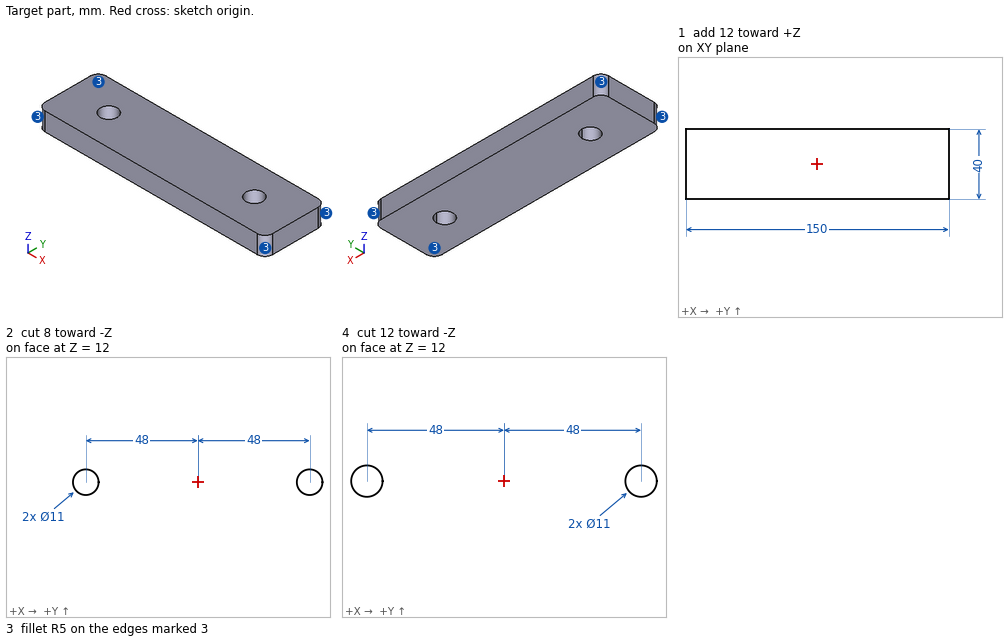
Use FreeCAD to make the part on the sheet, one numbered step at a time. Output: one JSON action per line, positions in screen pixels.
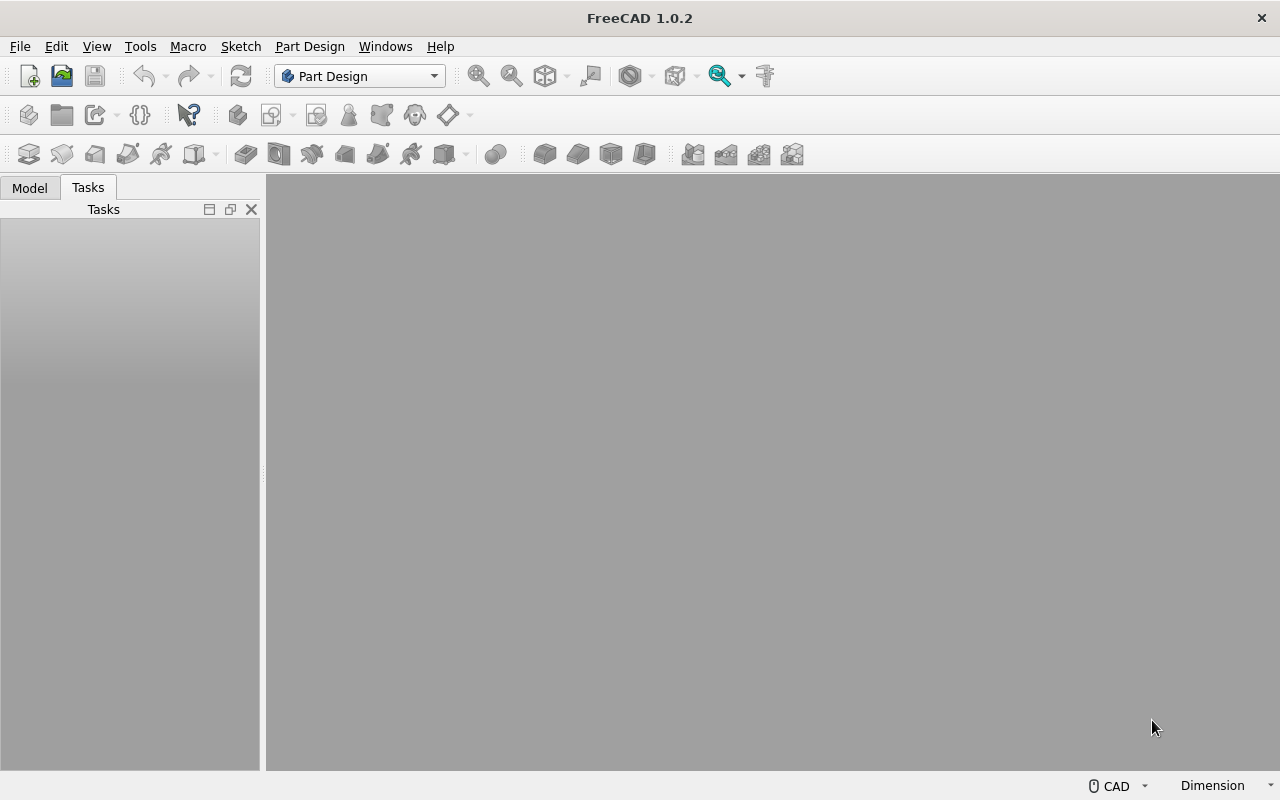
{"action": "left_click", "coordinate": [29, 76]}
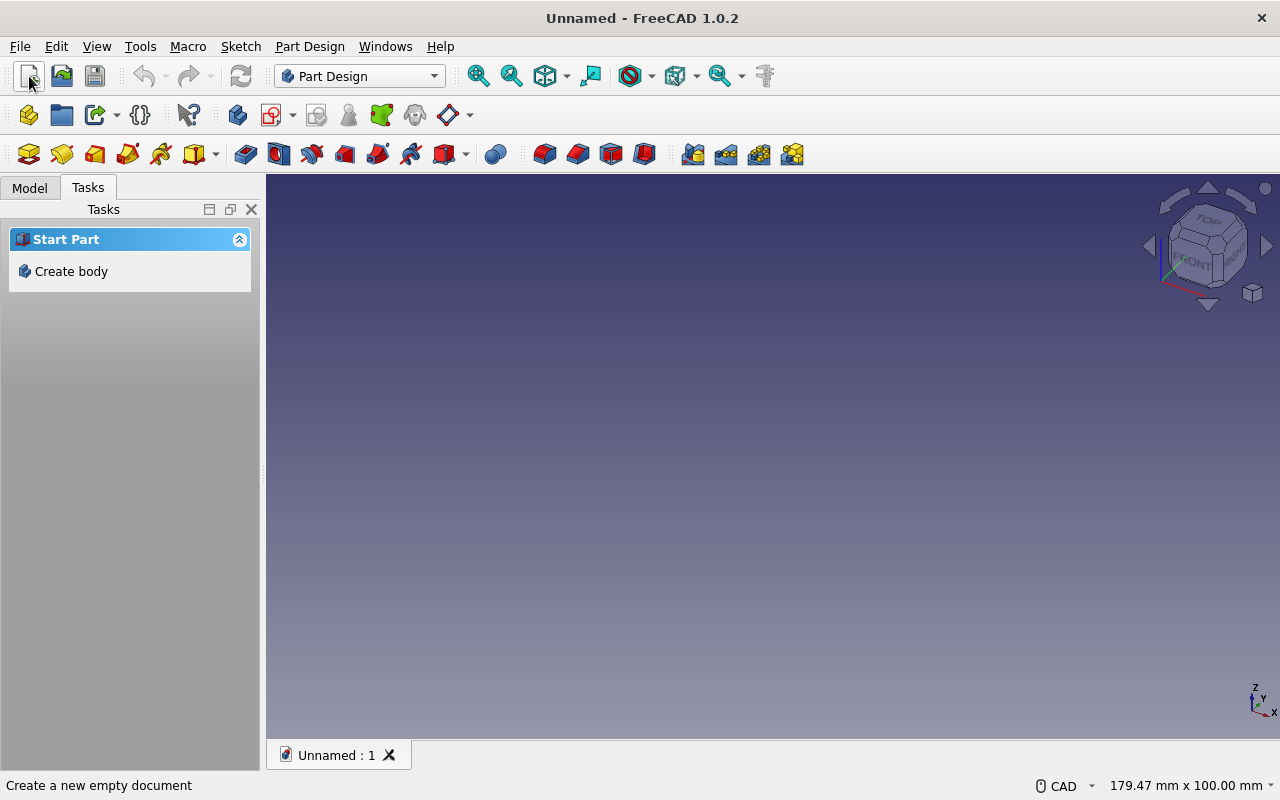
{"action": "left_click", "coordinate": [270, 116]}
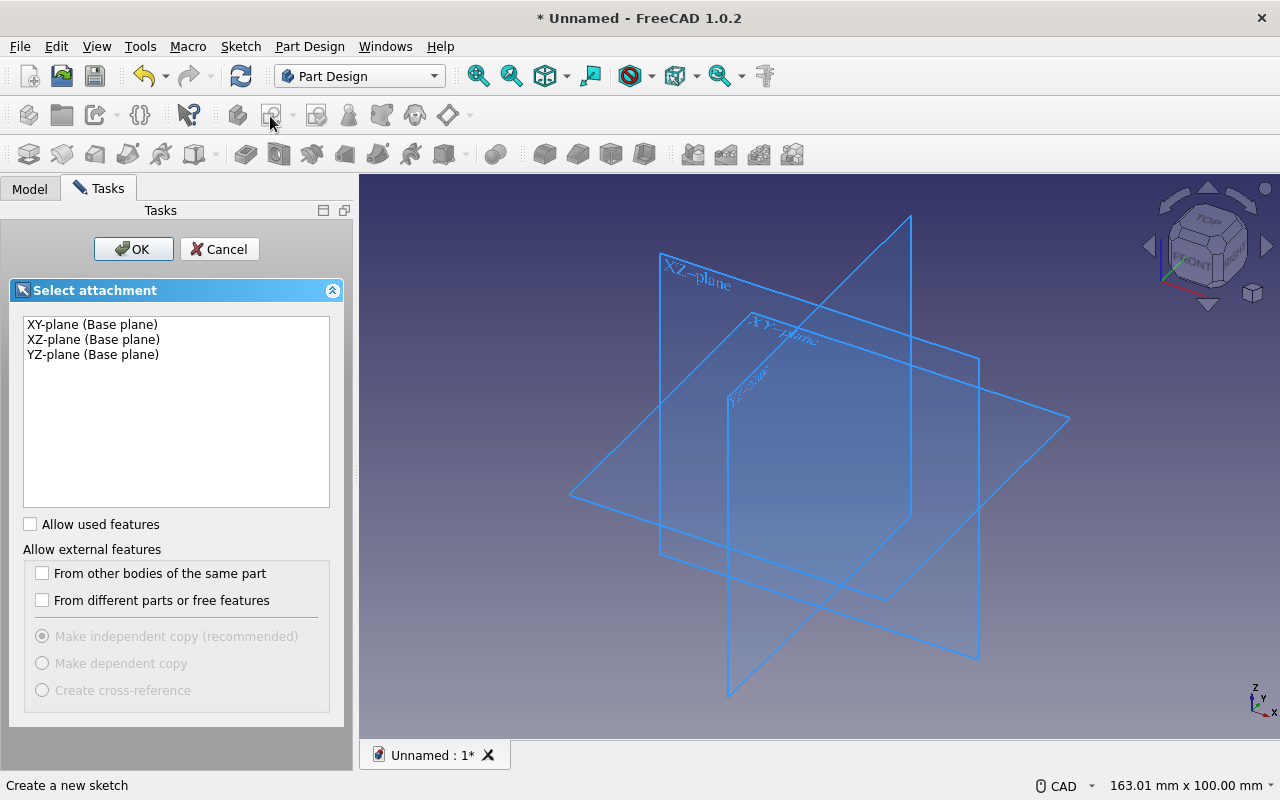
{"action": "left_click", "coordinate": [84, 324]}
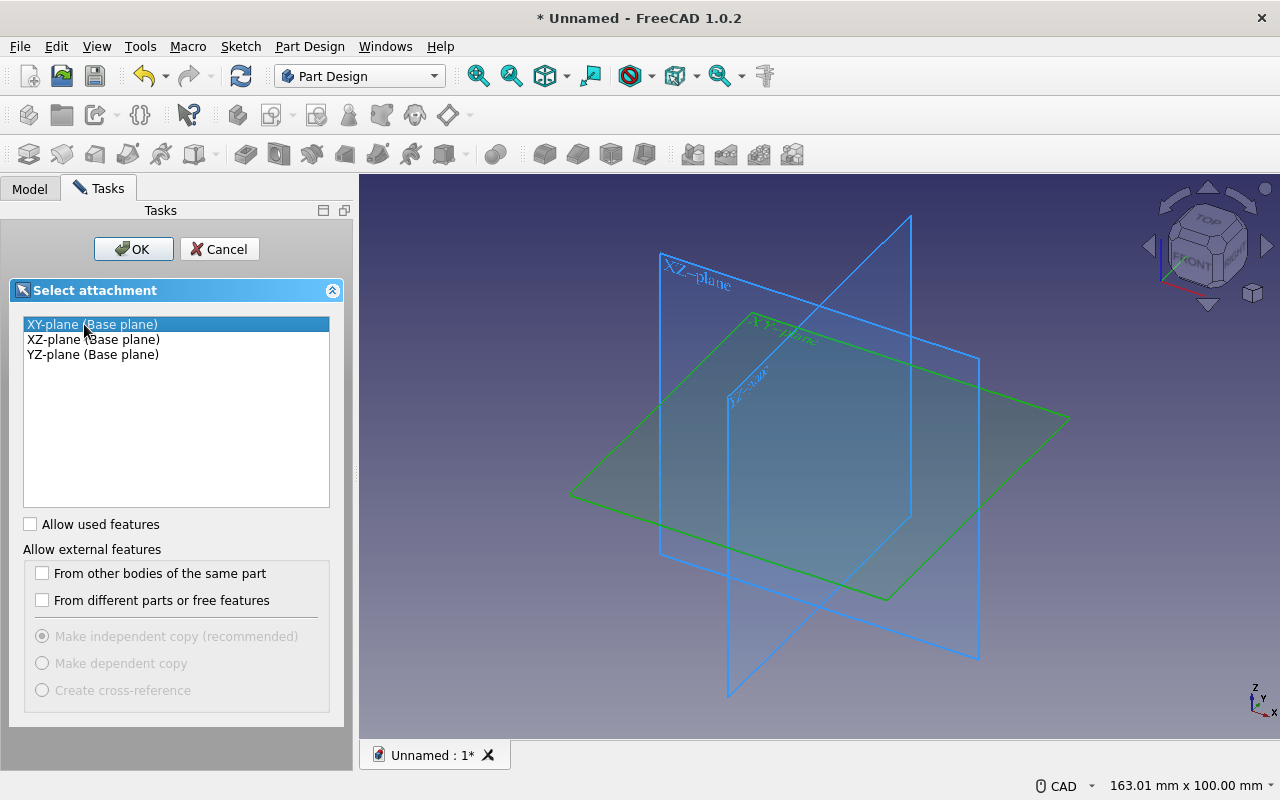
{"action": "left_click", "coordinate": [134, 249]}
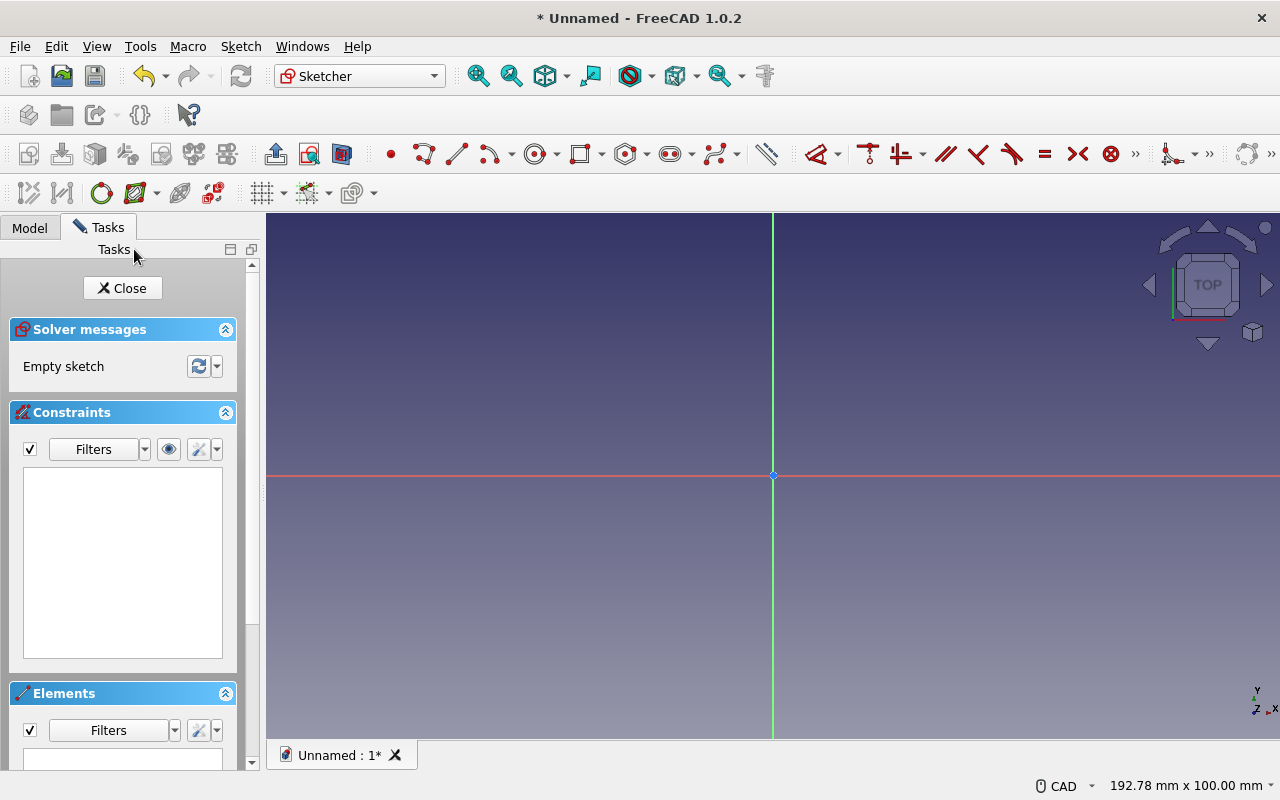
{"action": "scroll", "coordinate": [565, 476], "scroll_direction": "down", "scroll_amount": 2}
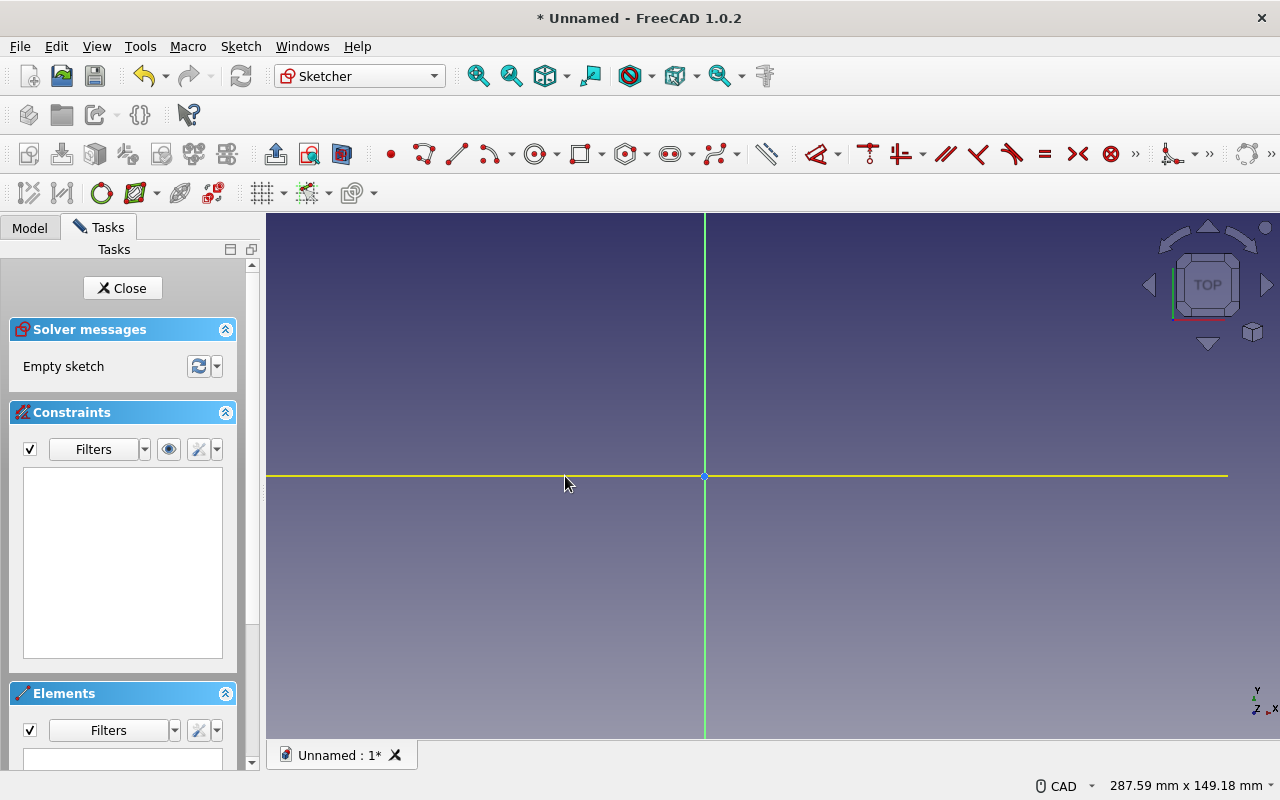
{"action": "left_click", "coordinate": [602, 154]}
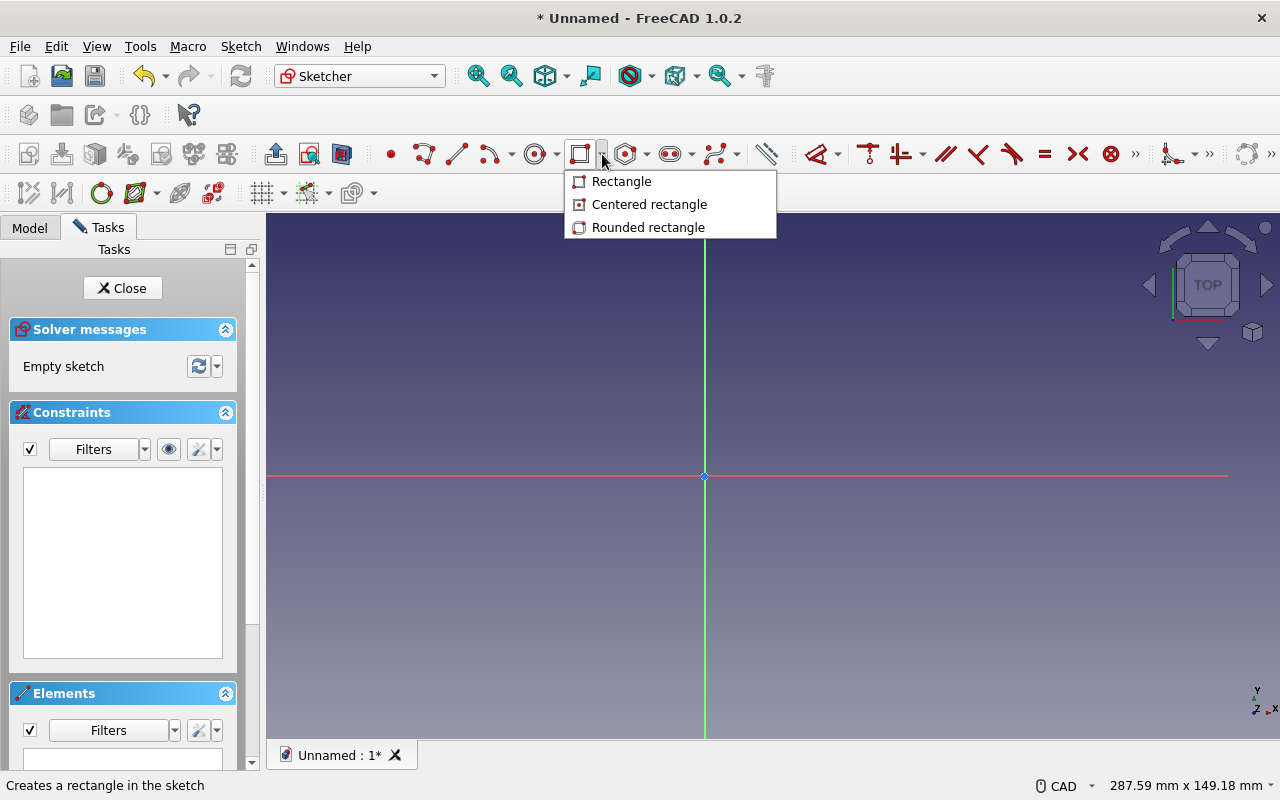
{"action": "left_click", "coordinate": [670, 204]}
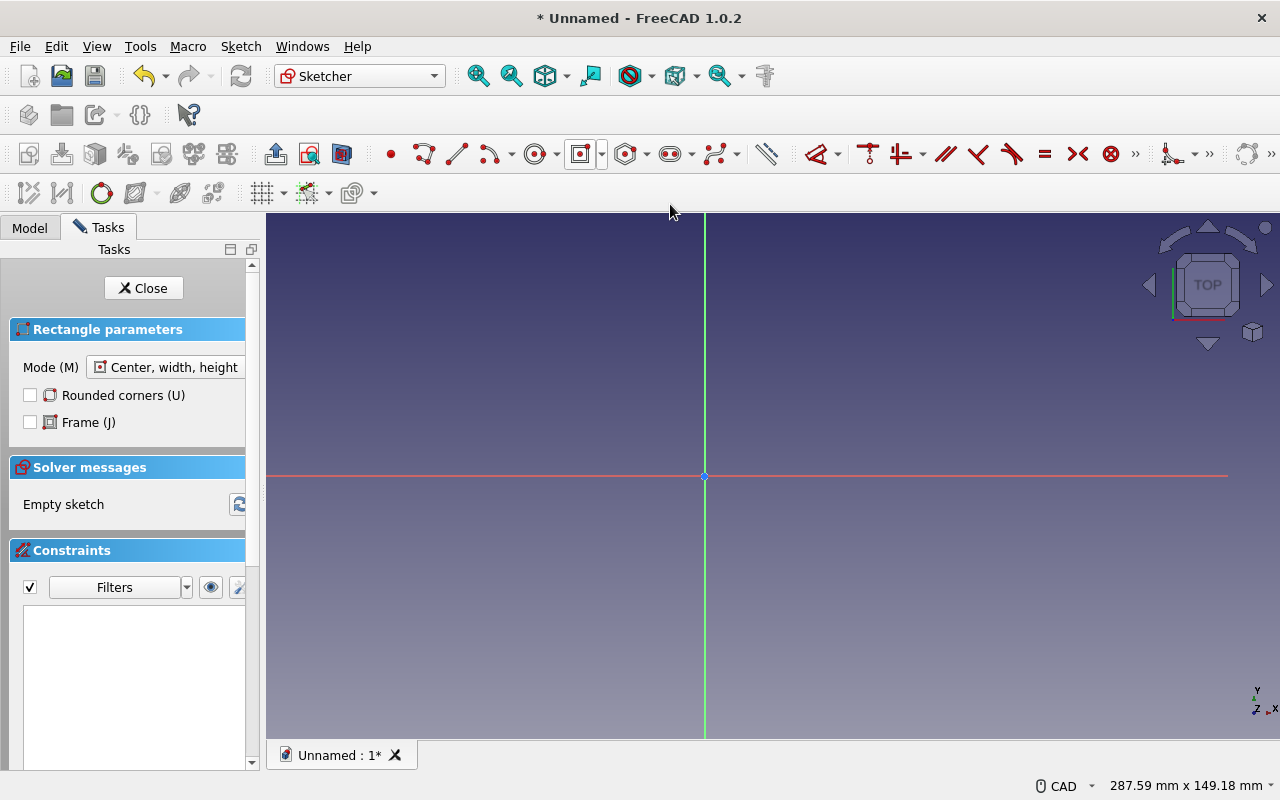
{"action": "left_click", "coordinate": [705, 476]}
{"action": "left_click", "coordinate": [969, 406]}
{"action": "key", "text": "Escape"}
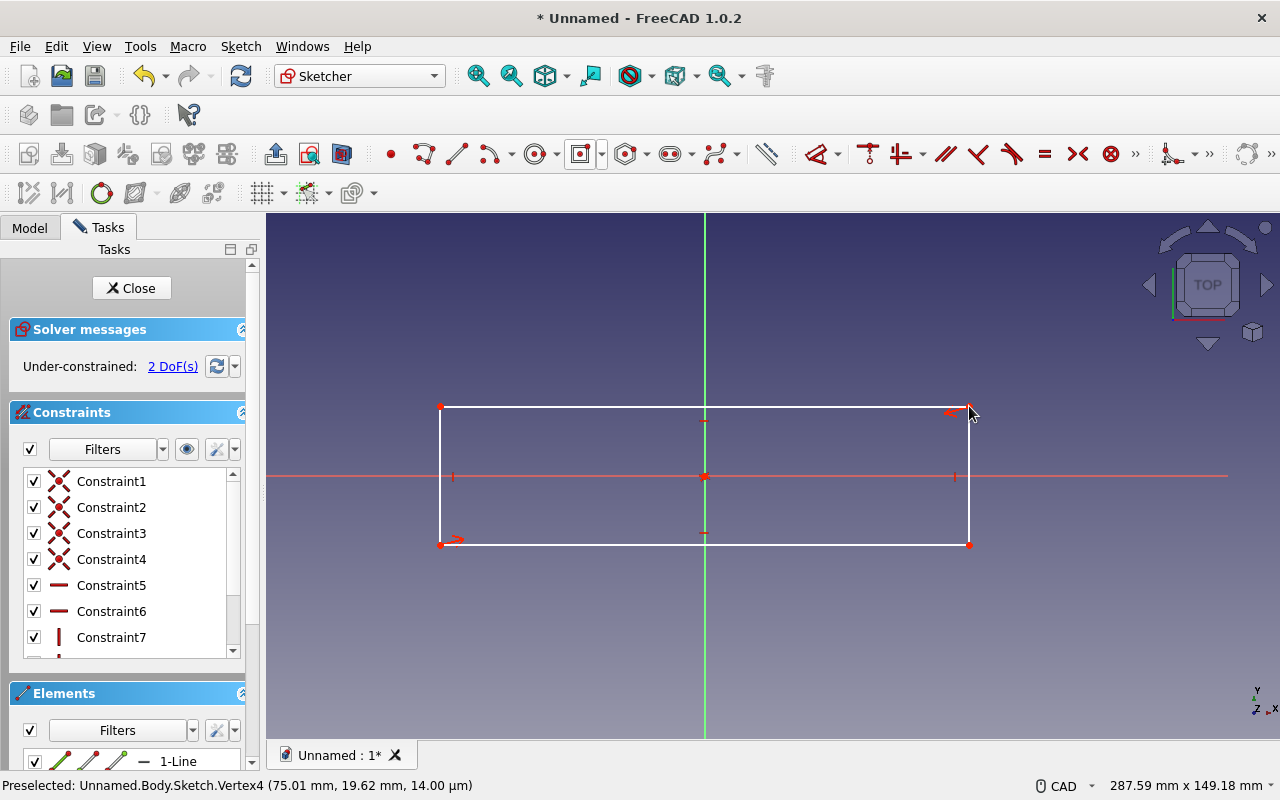
{"action": "left_click", "coordinate": [816, 154]}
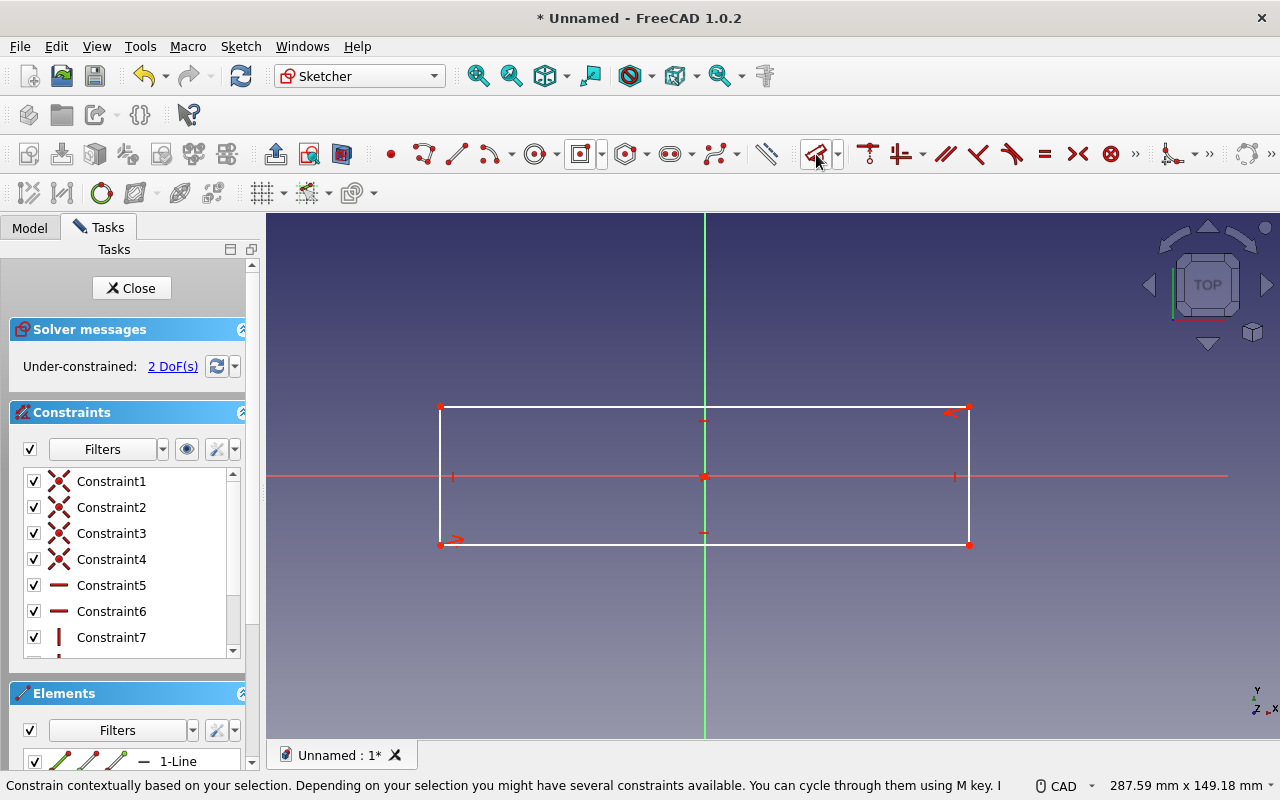
{"action": "left_click", "coordinate": [969, 504]}
{"action": "left_click", "coordinate": [1003, 444]}